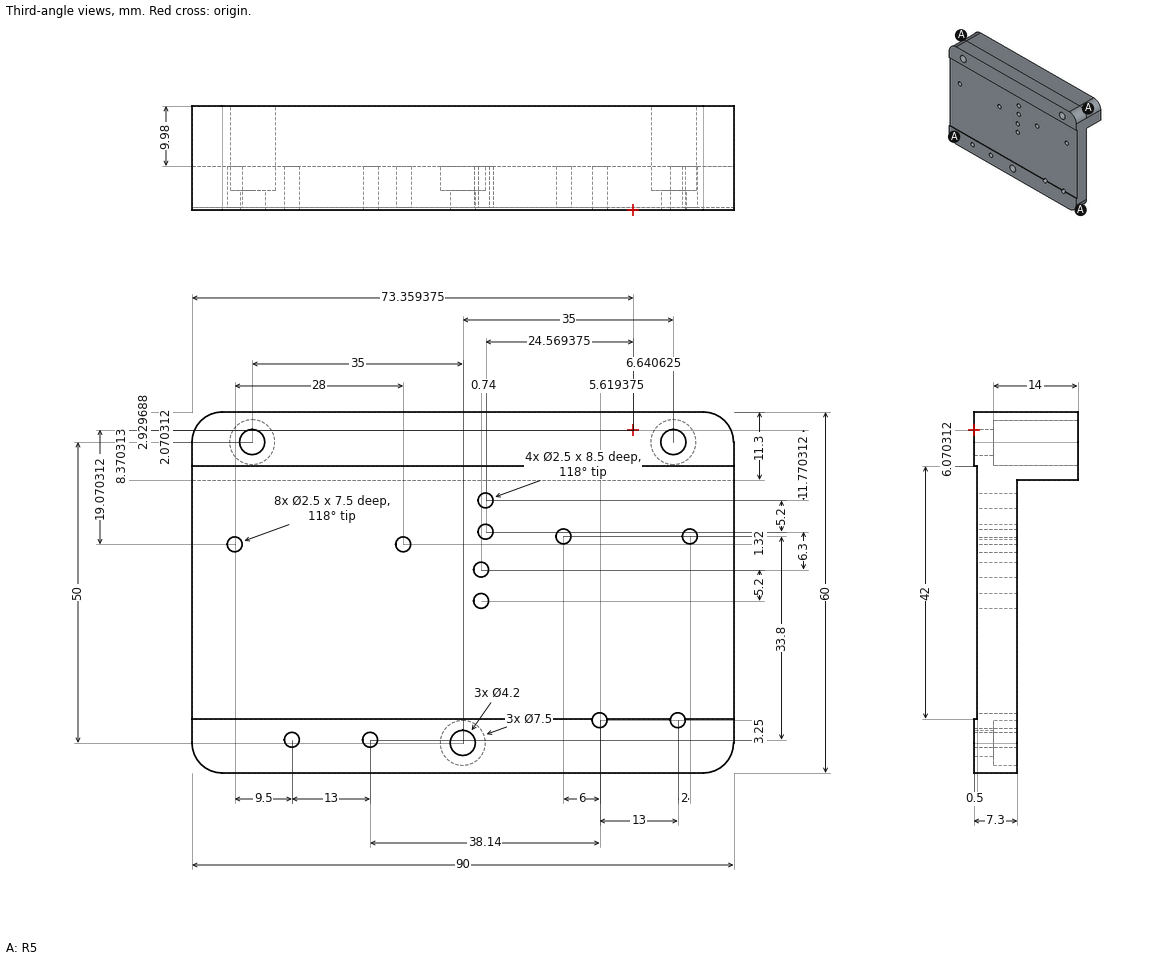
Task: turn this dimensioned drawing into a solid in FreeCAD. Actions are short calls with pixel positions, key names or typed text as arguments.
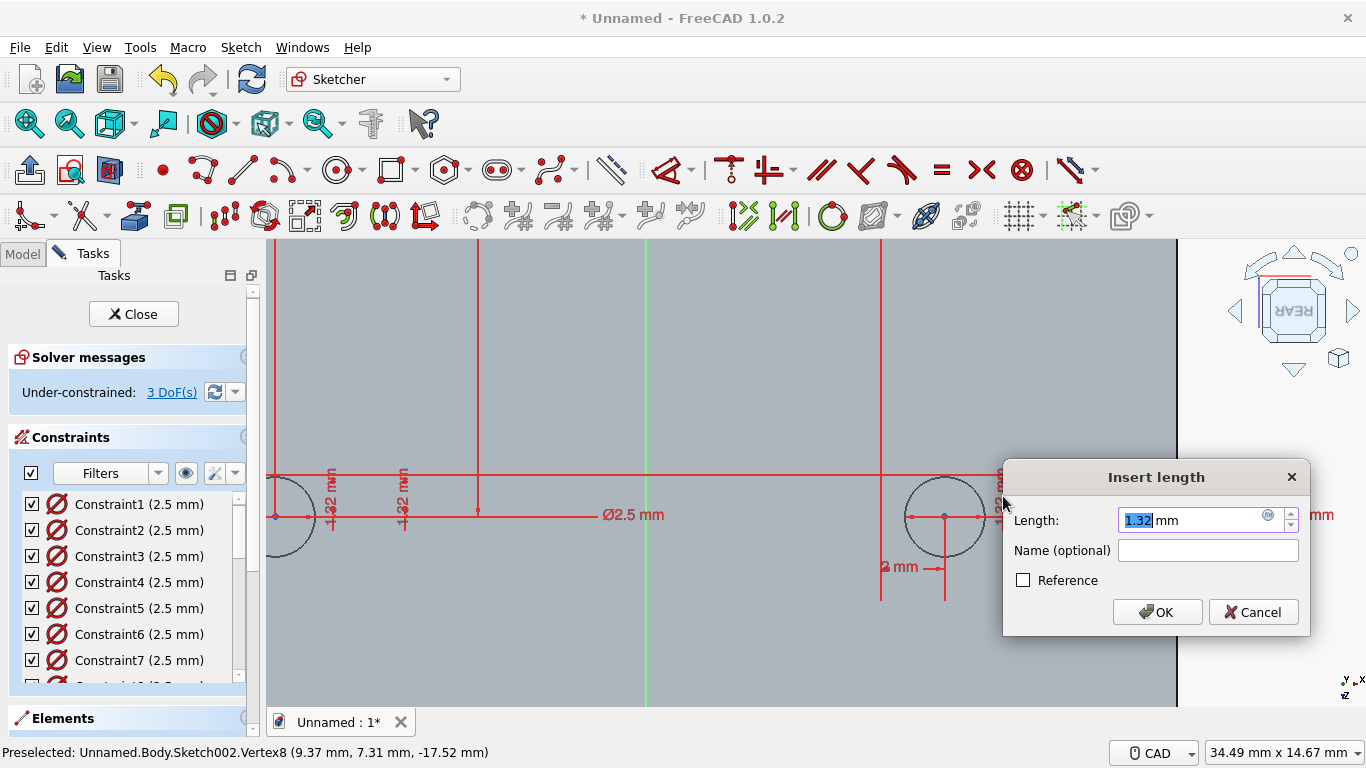
text(1.32)
key(Return)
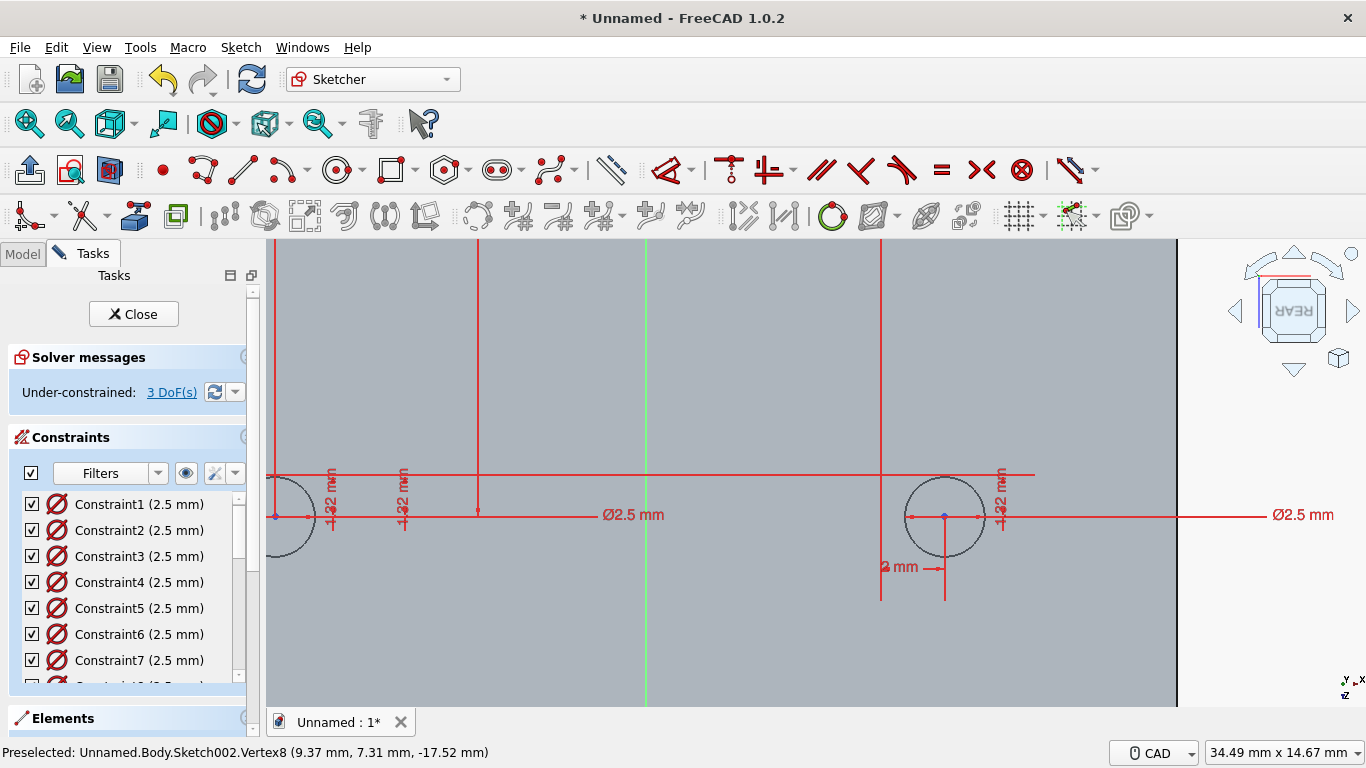
scroll(947, 520, down, 9)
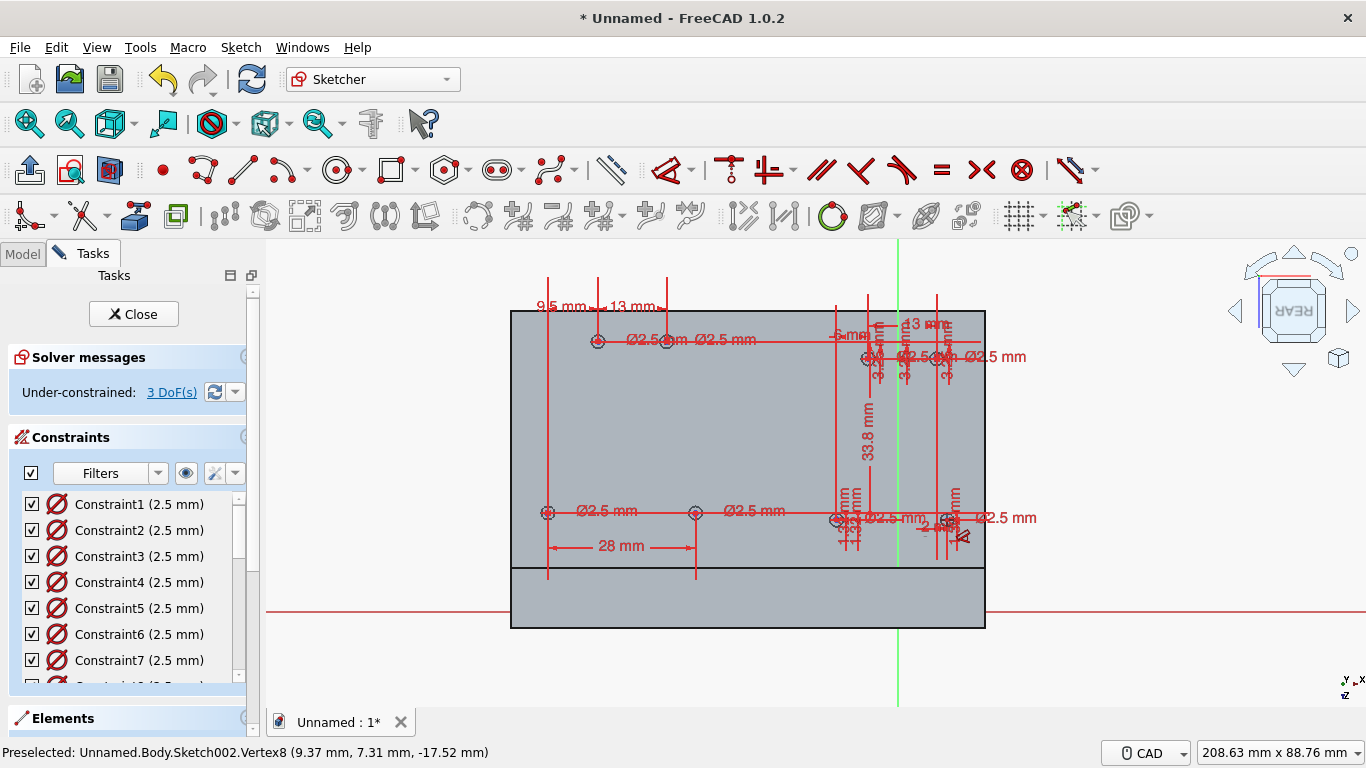
click(667, 342)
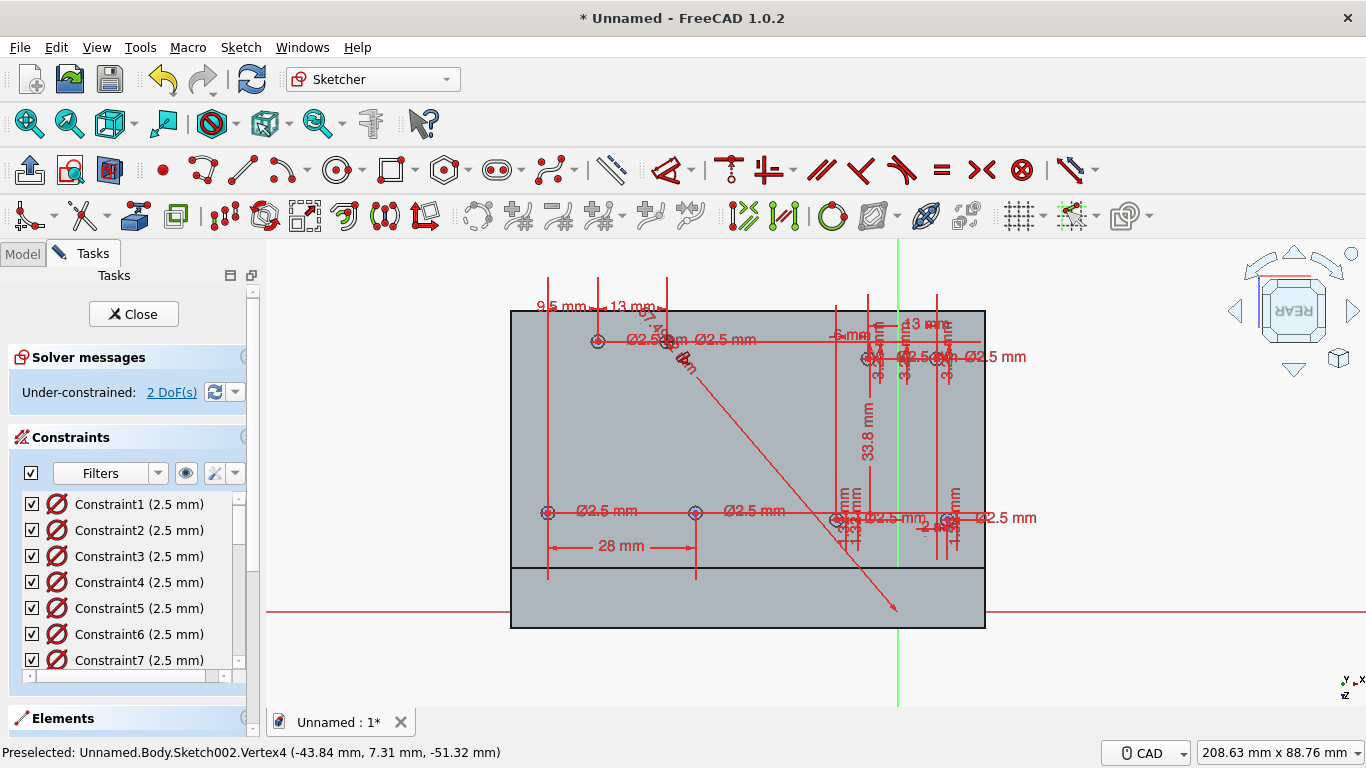
click(868, 359)
click(767, 308)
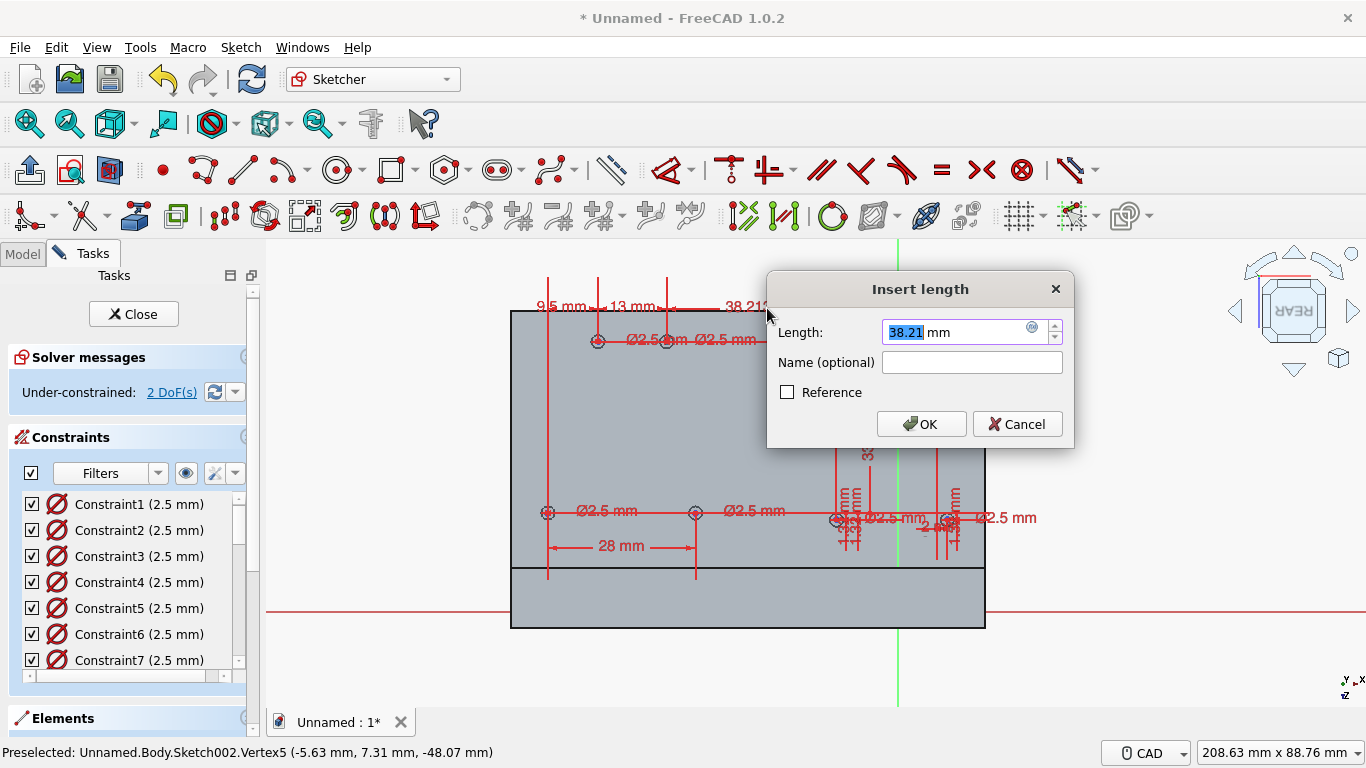
text(38.14)
key(Return)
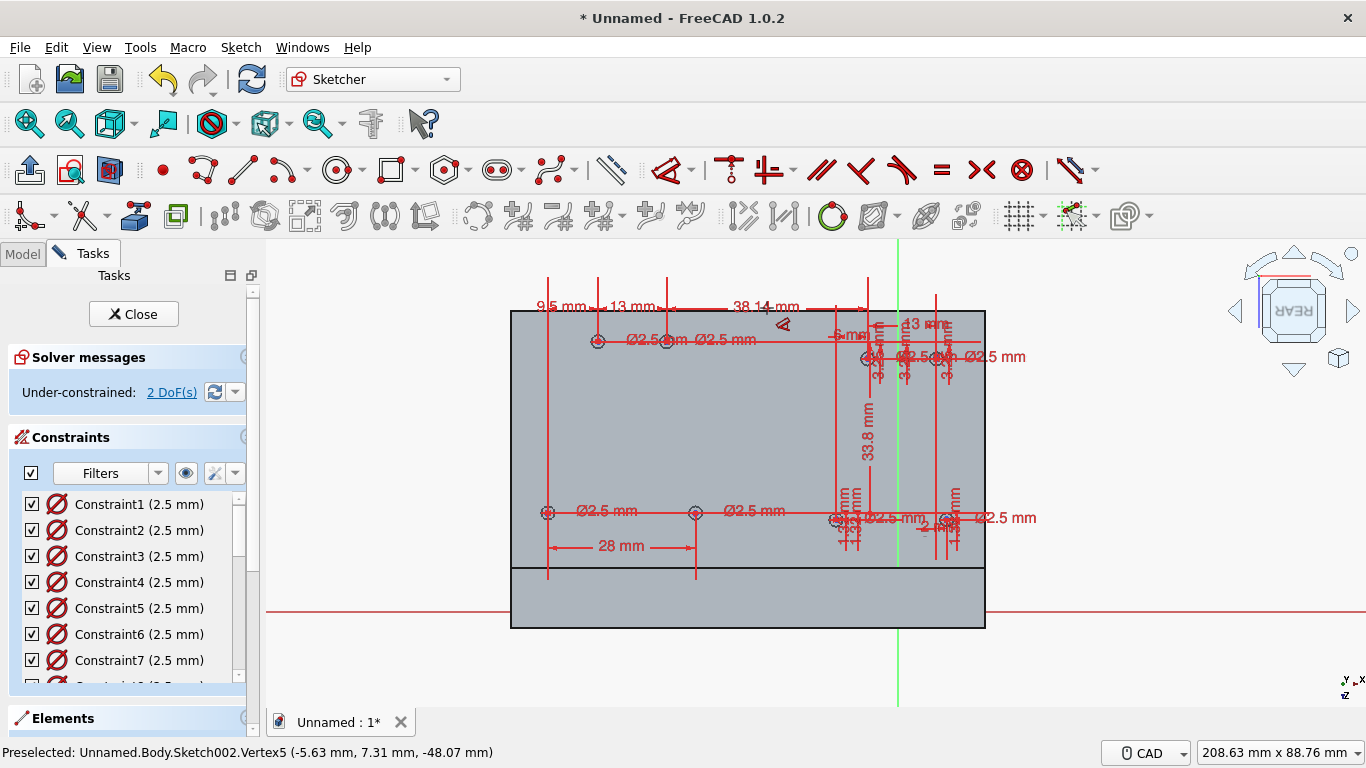
scroll(868, 359, up, 2)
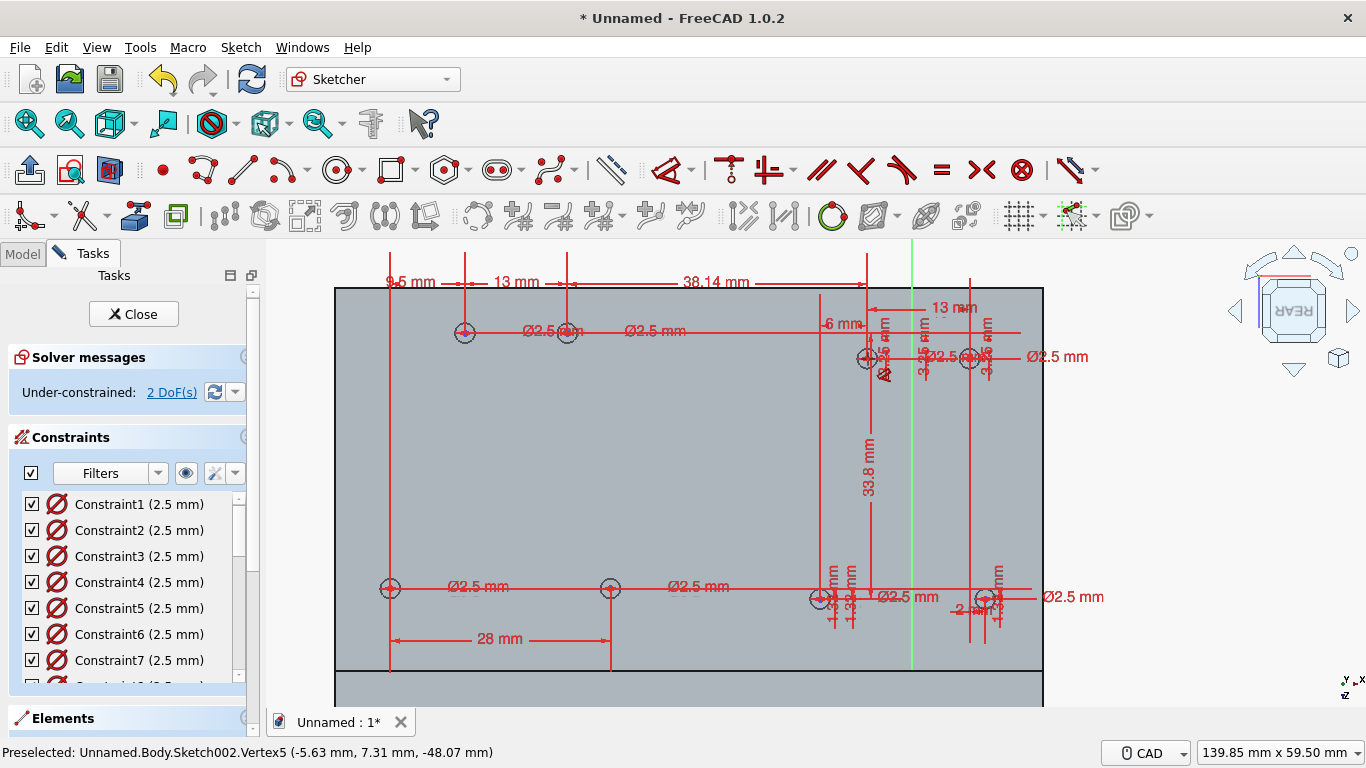
click(867, 359)
click(879, 301)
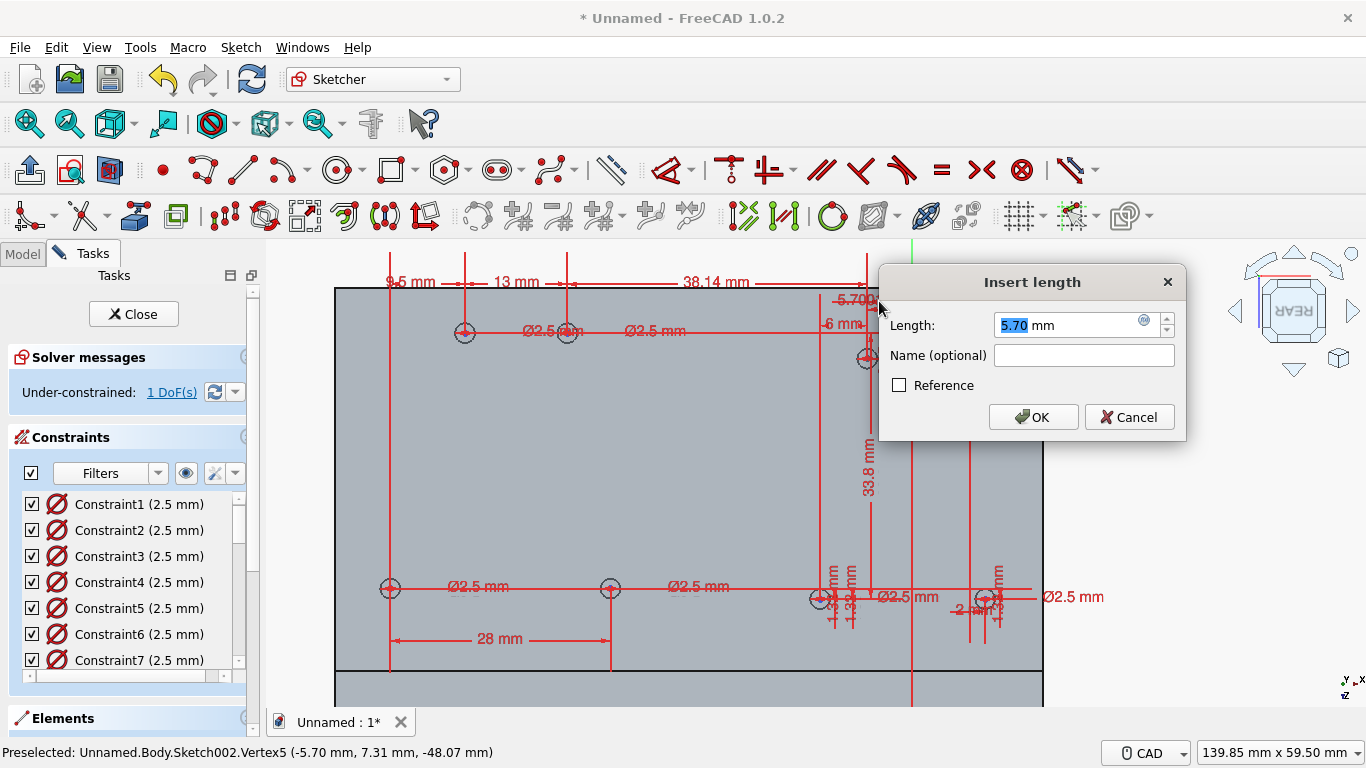
text(5.619375)
key(Return)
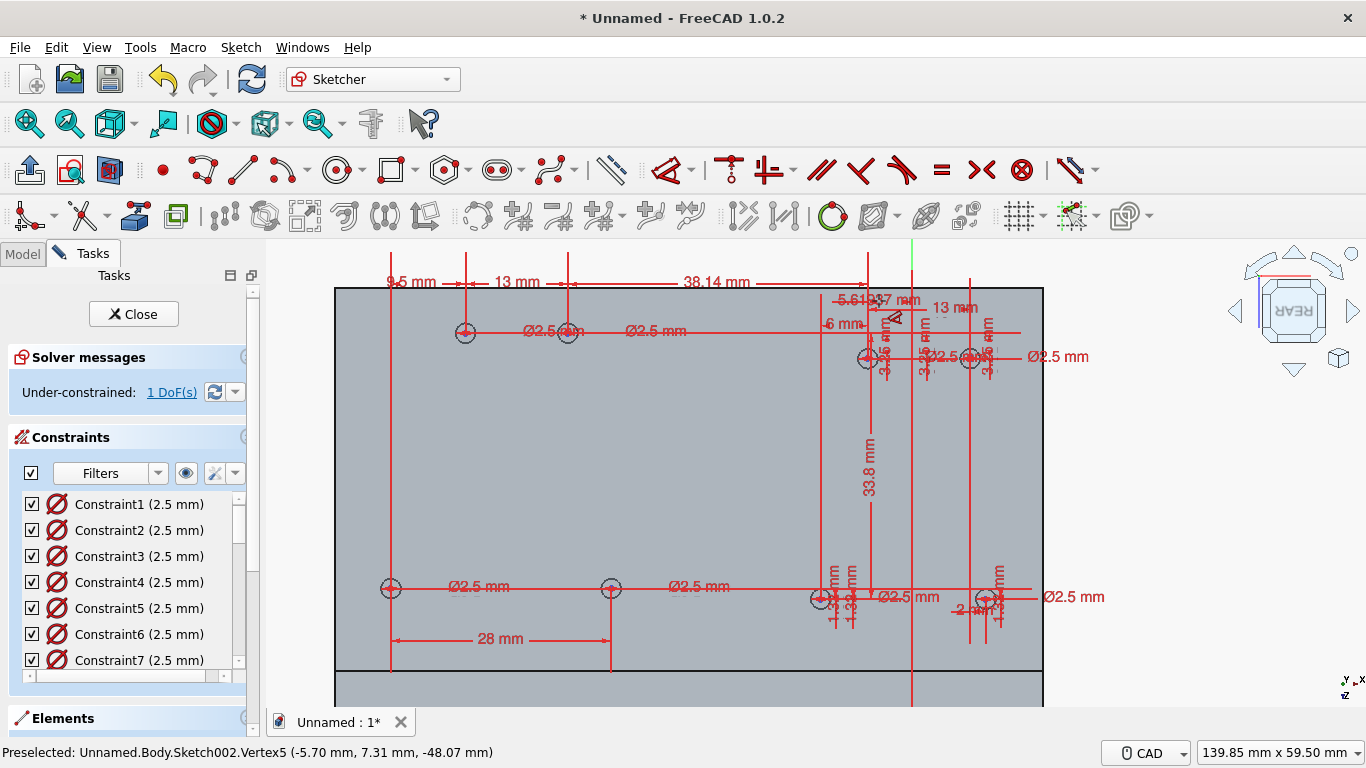
click(391, 589)
click(357, 634)